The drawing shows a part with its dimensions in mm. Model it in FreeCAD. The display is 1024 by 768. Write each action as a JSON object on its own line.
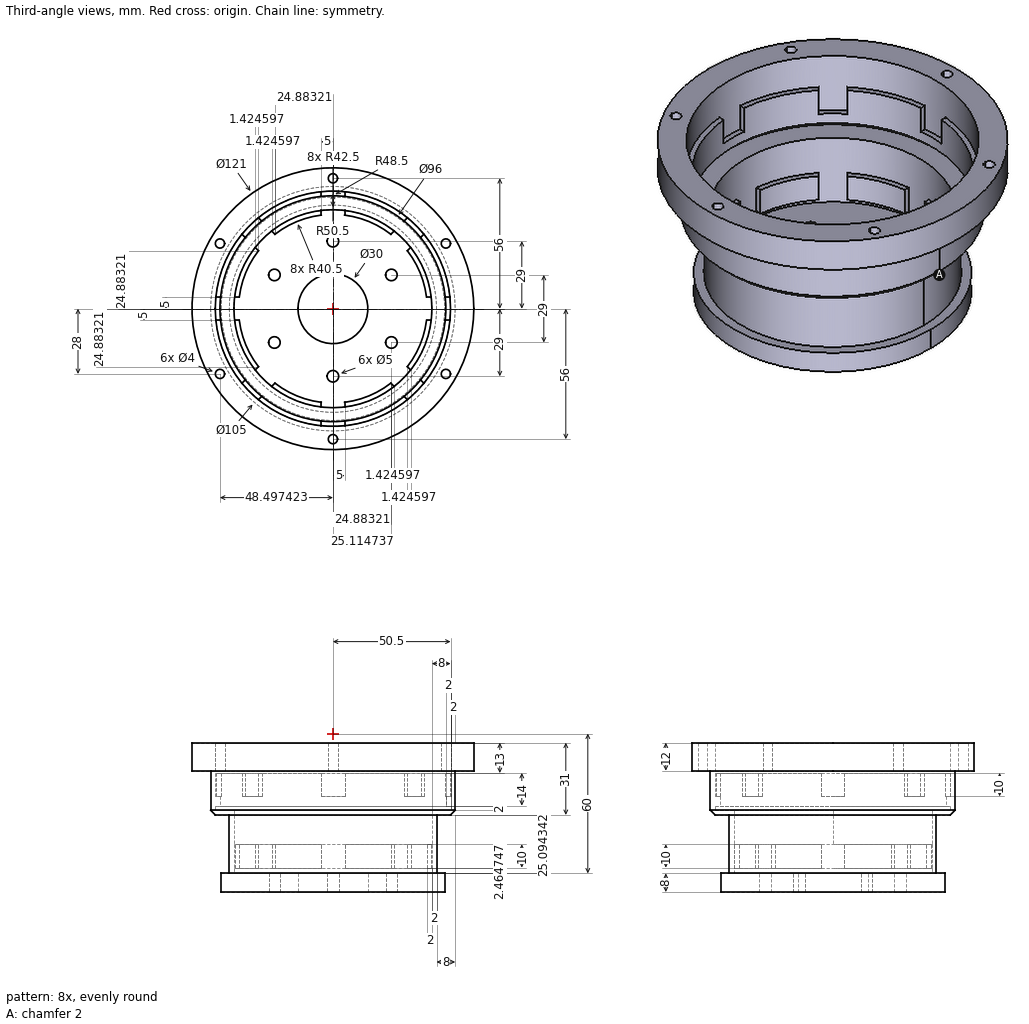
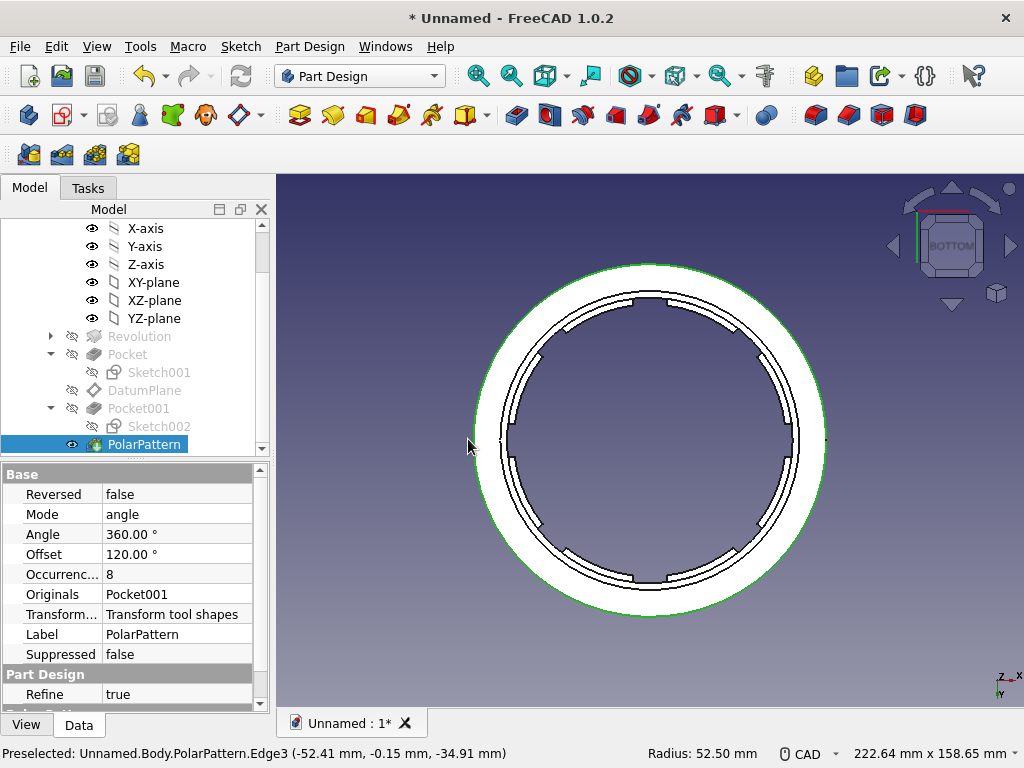
{"action": "left_click", "coordinate": [849, 116]}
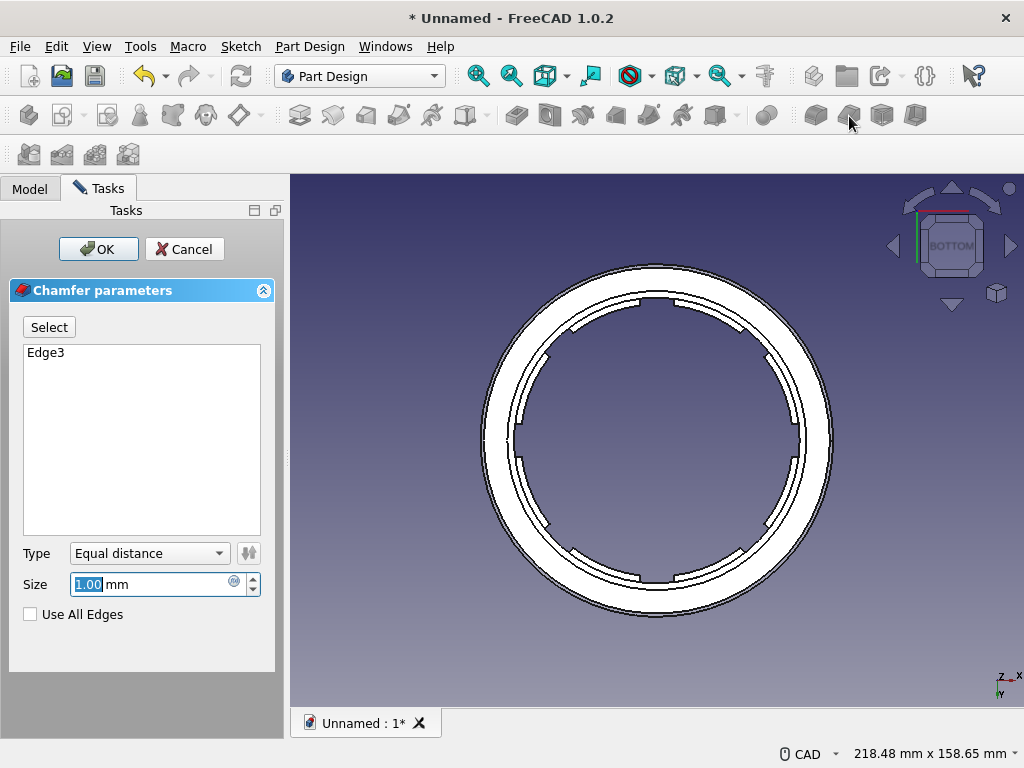
{"action": "type", "text": "2"}
{"action": "key", "text": "Tab"}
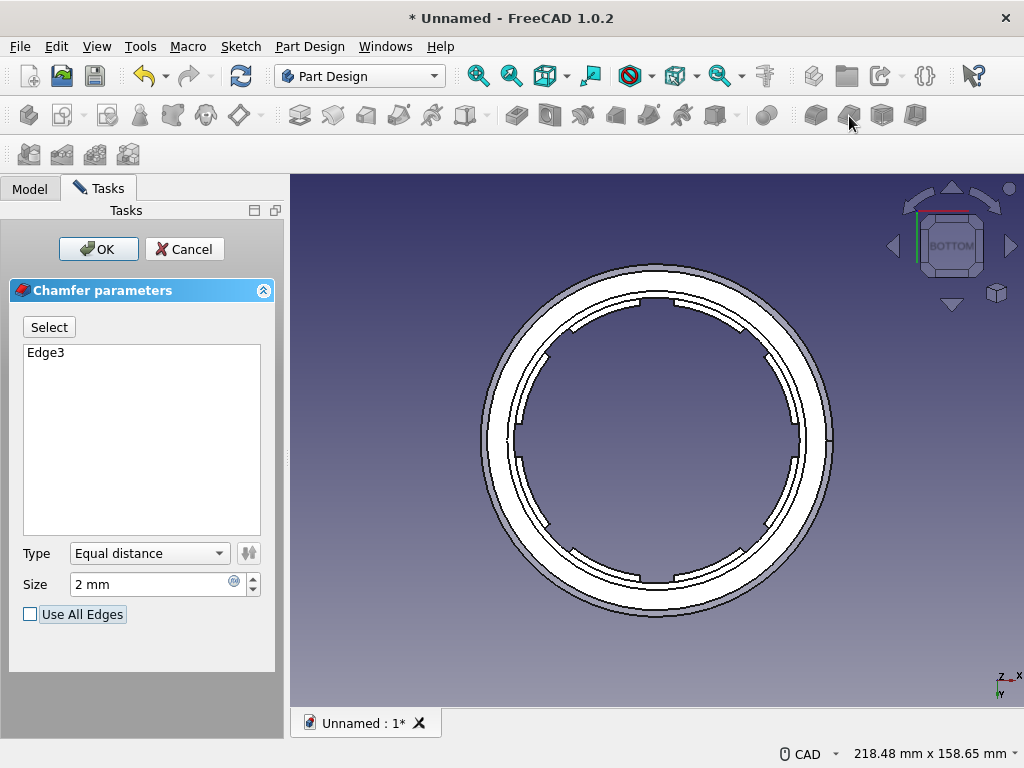
{"action": "left_click", "coordinate": [99, 249]}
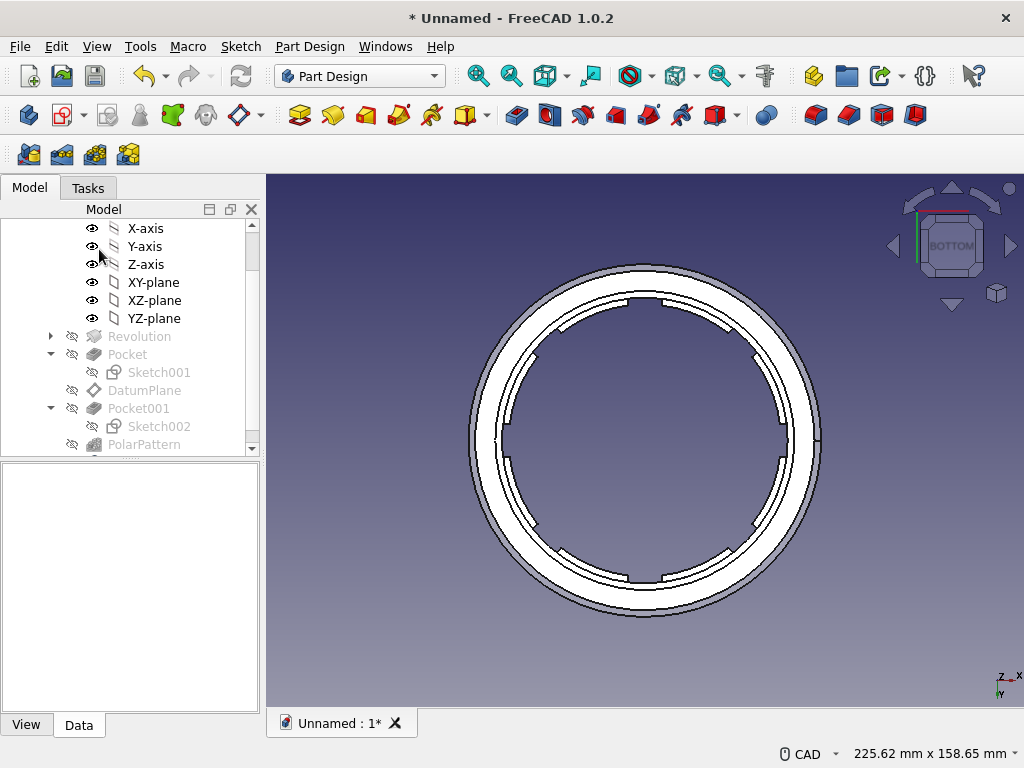
{"action": "scroll", "coordinate": [644, 587], "scroll_direction": "up", "scroll_amount": 9}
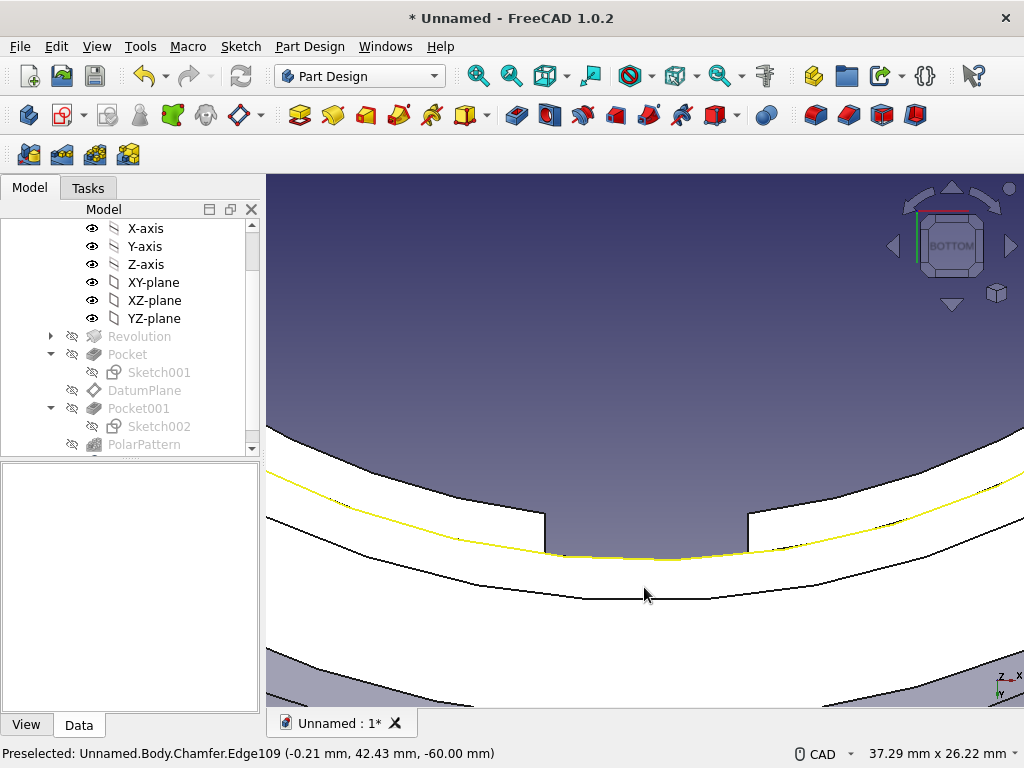
{"action": "left_click", "coordinate": [639, 586]}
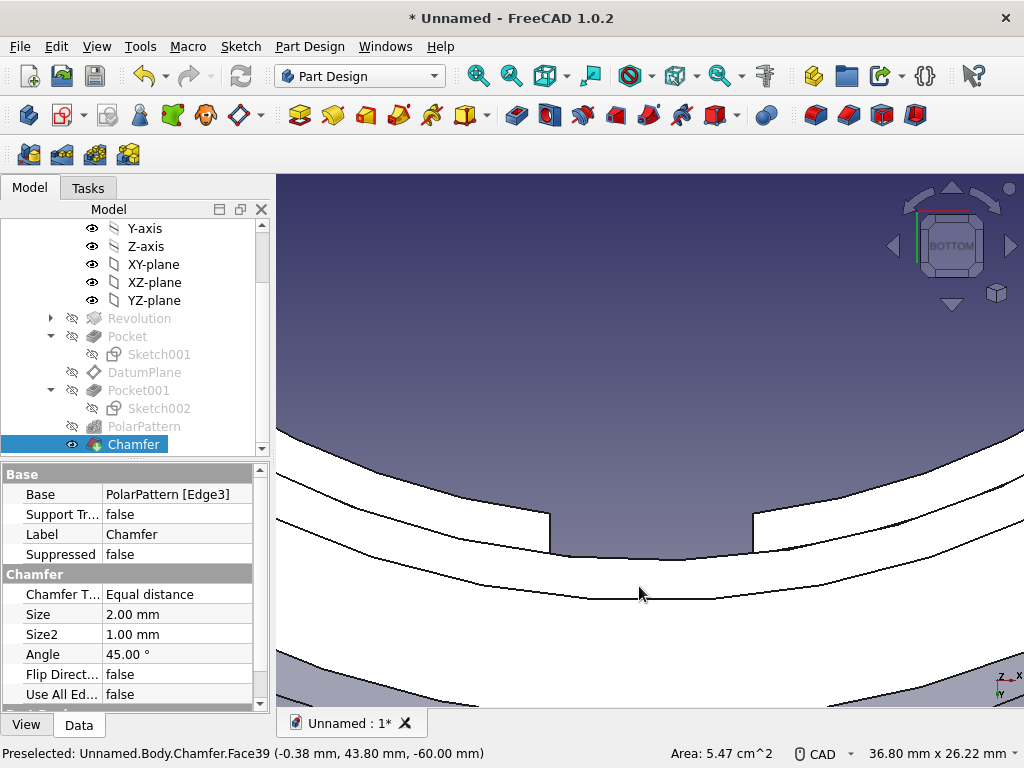
{"action": "left_click", "coordinate": [62, 116]}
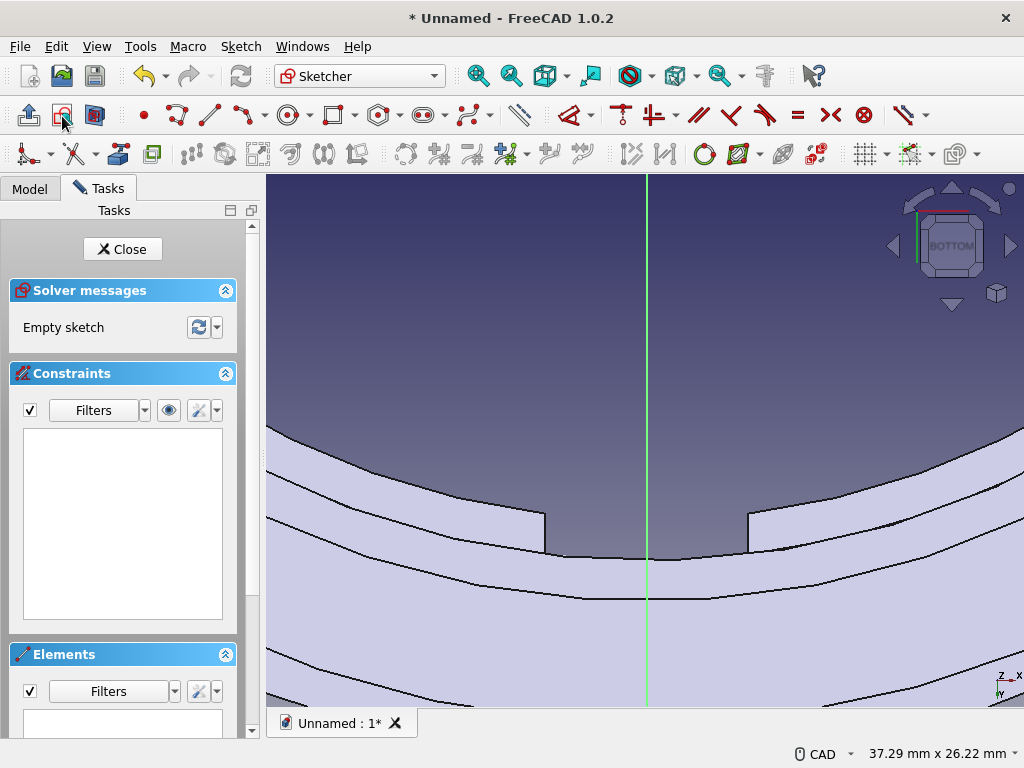
{"action": "scroll", "coordinate": [563, 588], "scroll_direction": "down", "scroll_amount": 9}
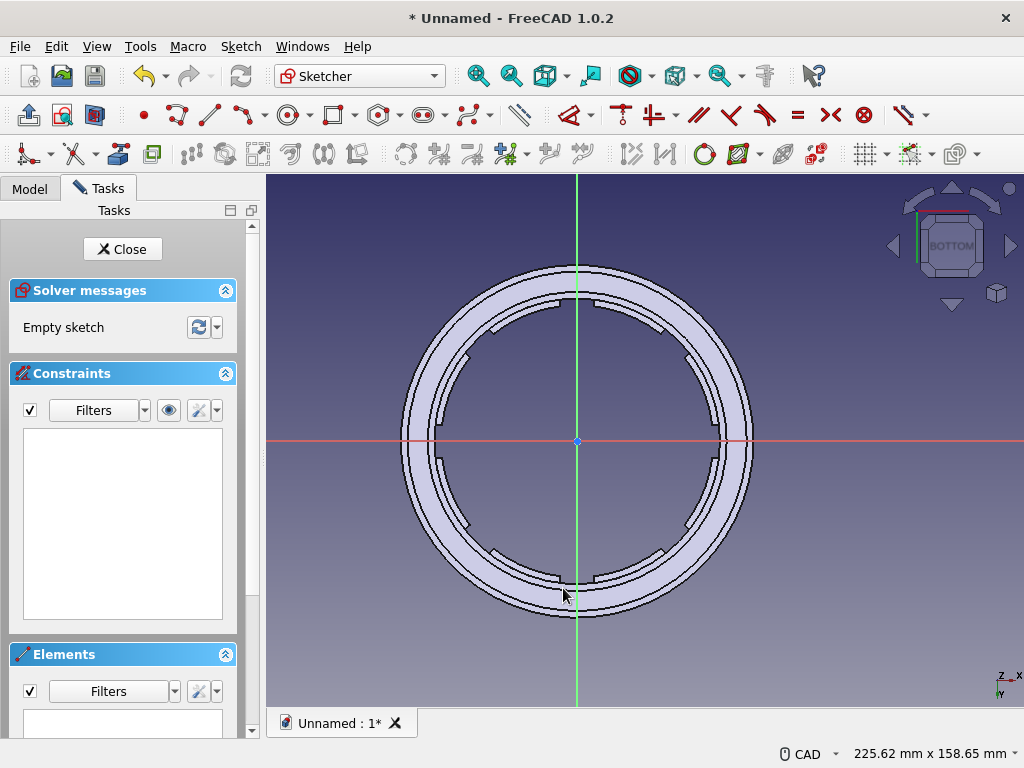
{"action": "key", "text": "g c"}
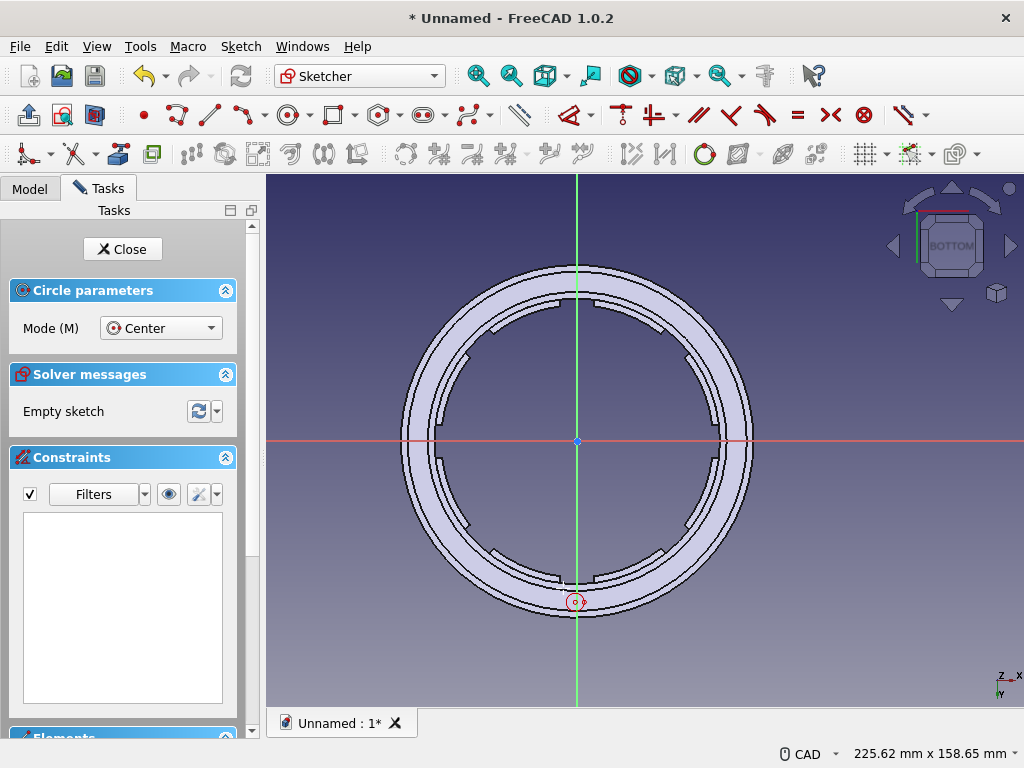
{"action": "left_click", "coordinate": [577, 441]}
{"action": "left_click", "coordinate": [691, 327]}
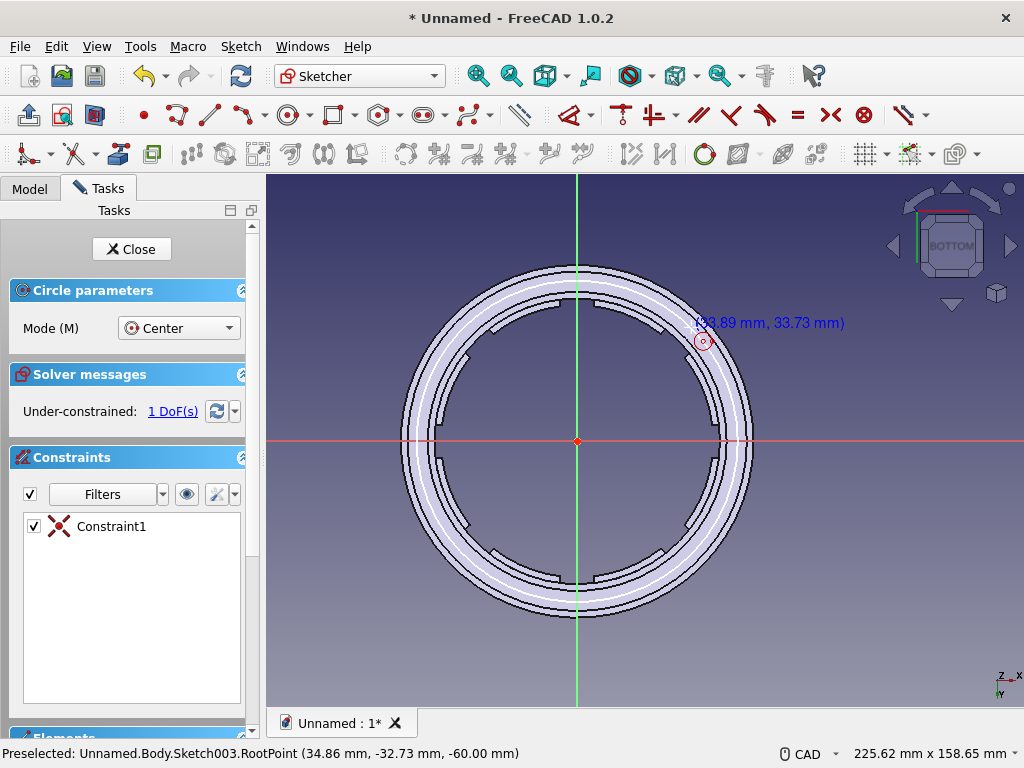
{"action": "scroll", "coordinate": [577, 344], "scroll_direction": "up", "scroll_amount": 5}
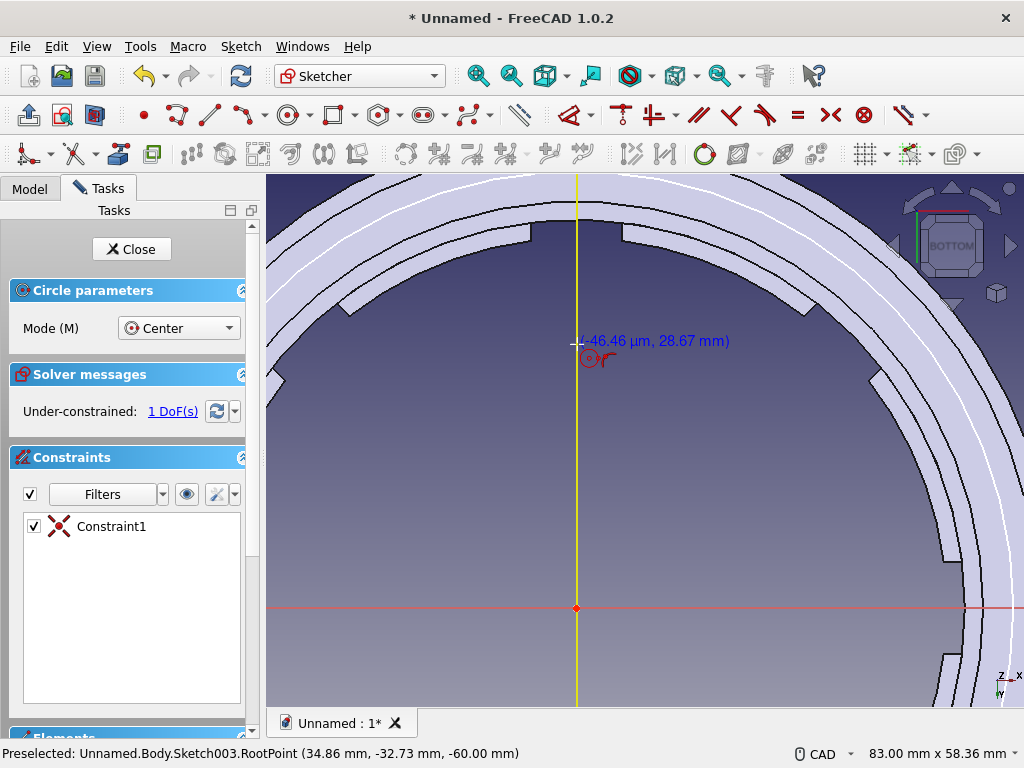
{"action": "left_click", "coordinate": [577, 343]}
{"action": "left_click", "coordinate": [593, 327]}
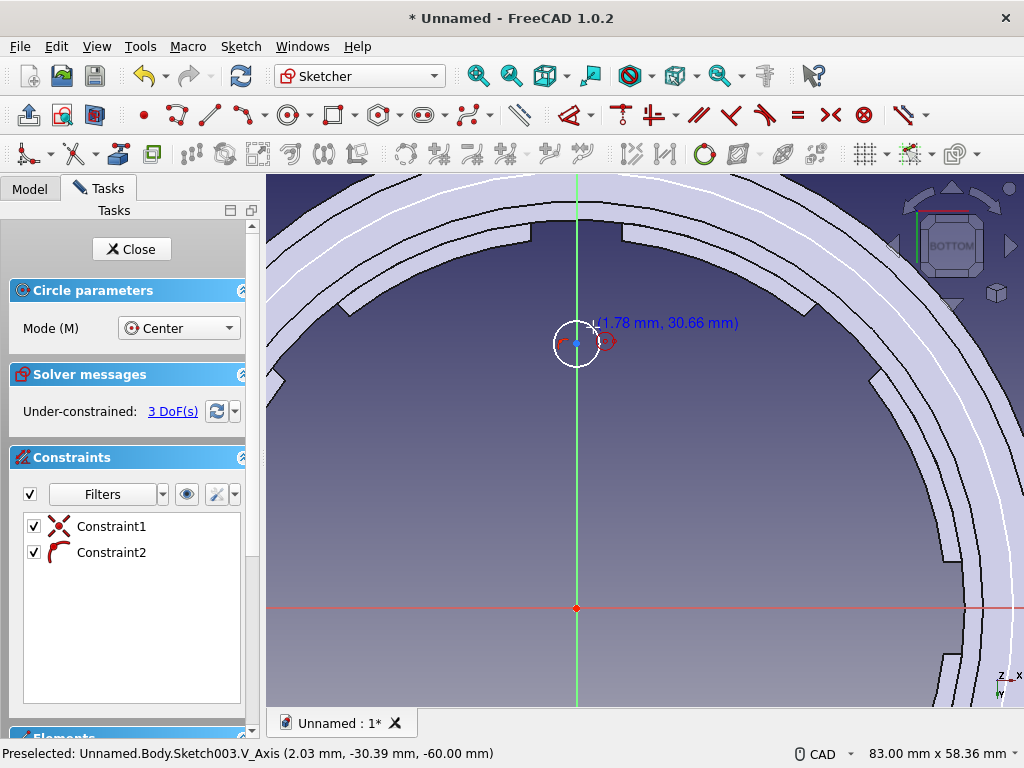
{"action": "left_click", "coordinate": [806, 476]}
{"action": "left_click", "coordinate": [822, 459]}